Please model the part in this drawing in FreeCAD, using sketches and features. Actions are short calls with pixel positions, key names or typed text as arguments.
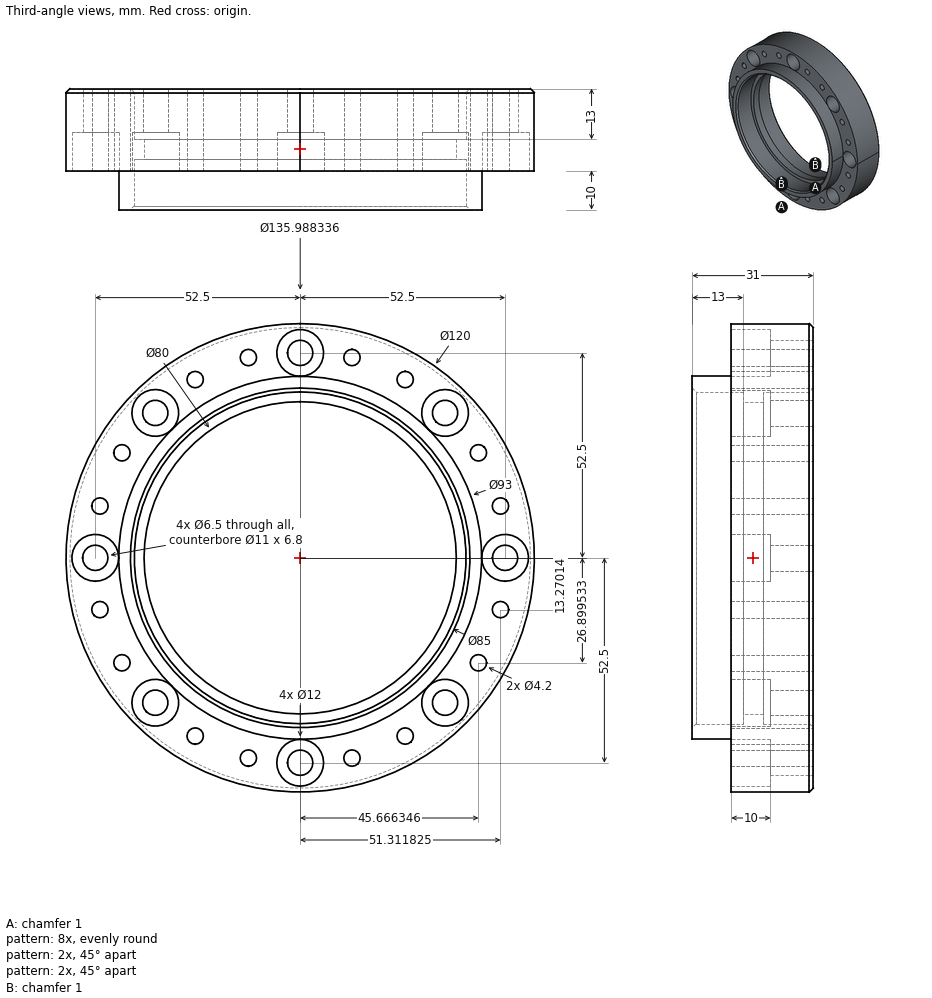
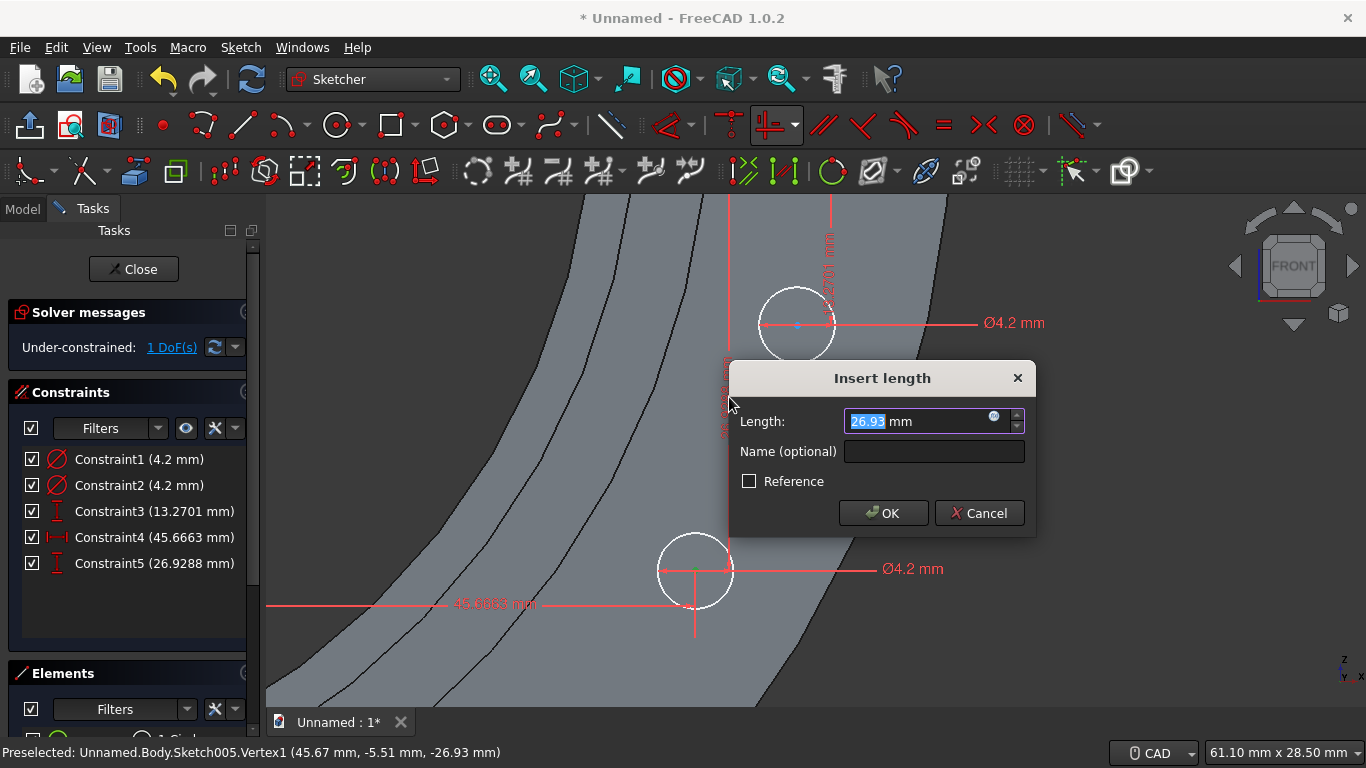
text(26.899533)
key(Return)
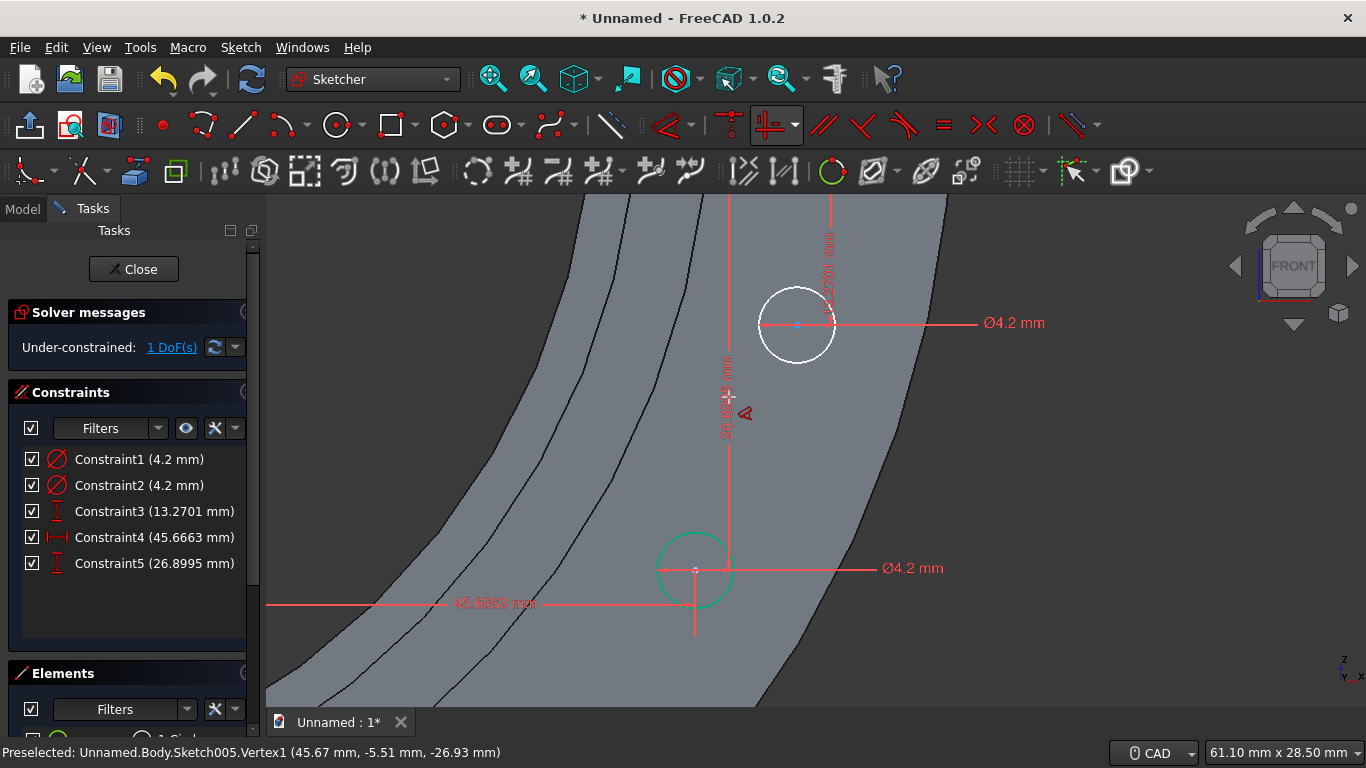
click(797, 325)
click(545, 359)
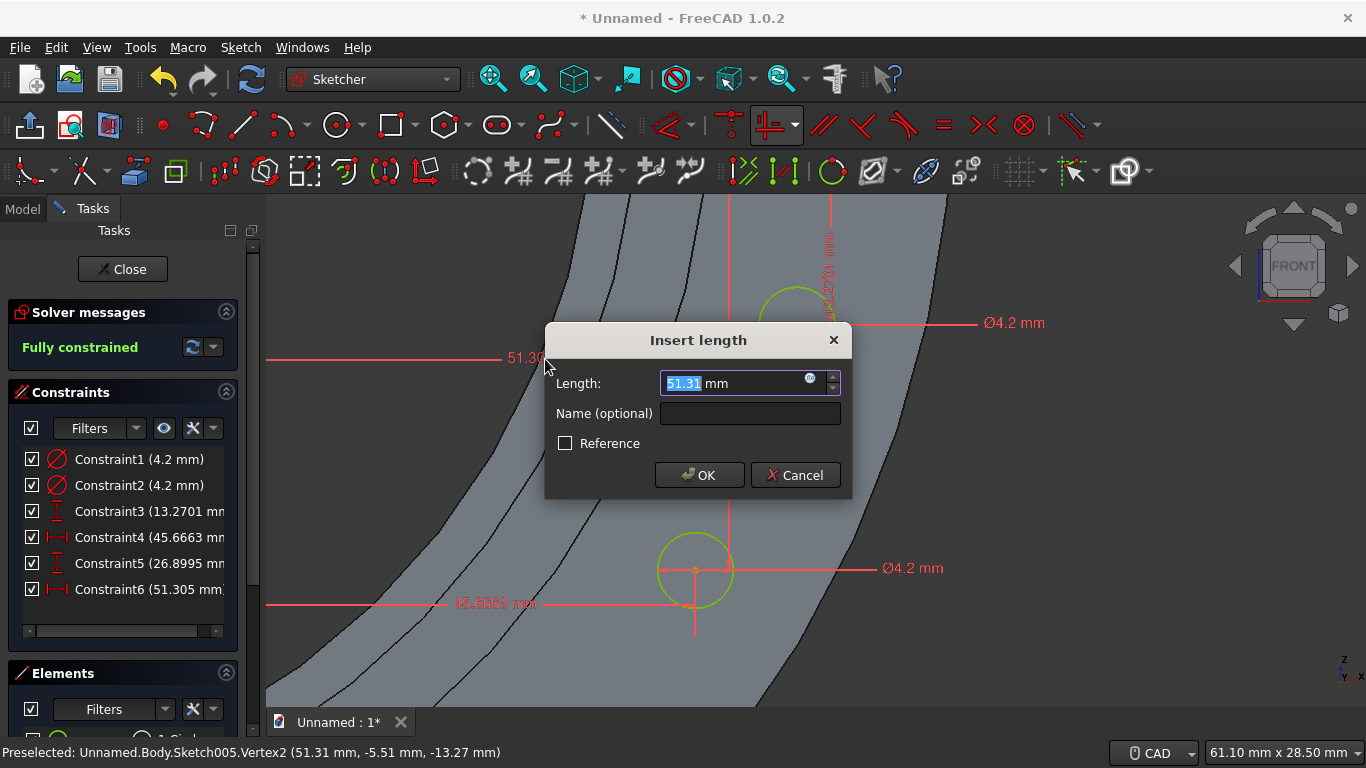
text(51.311825)
key(Return)
key(Escape)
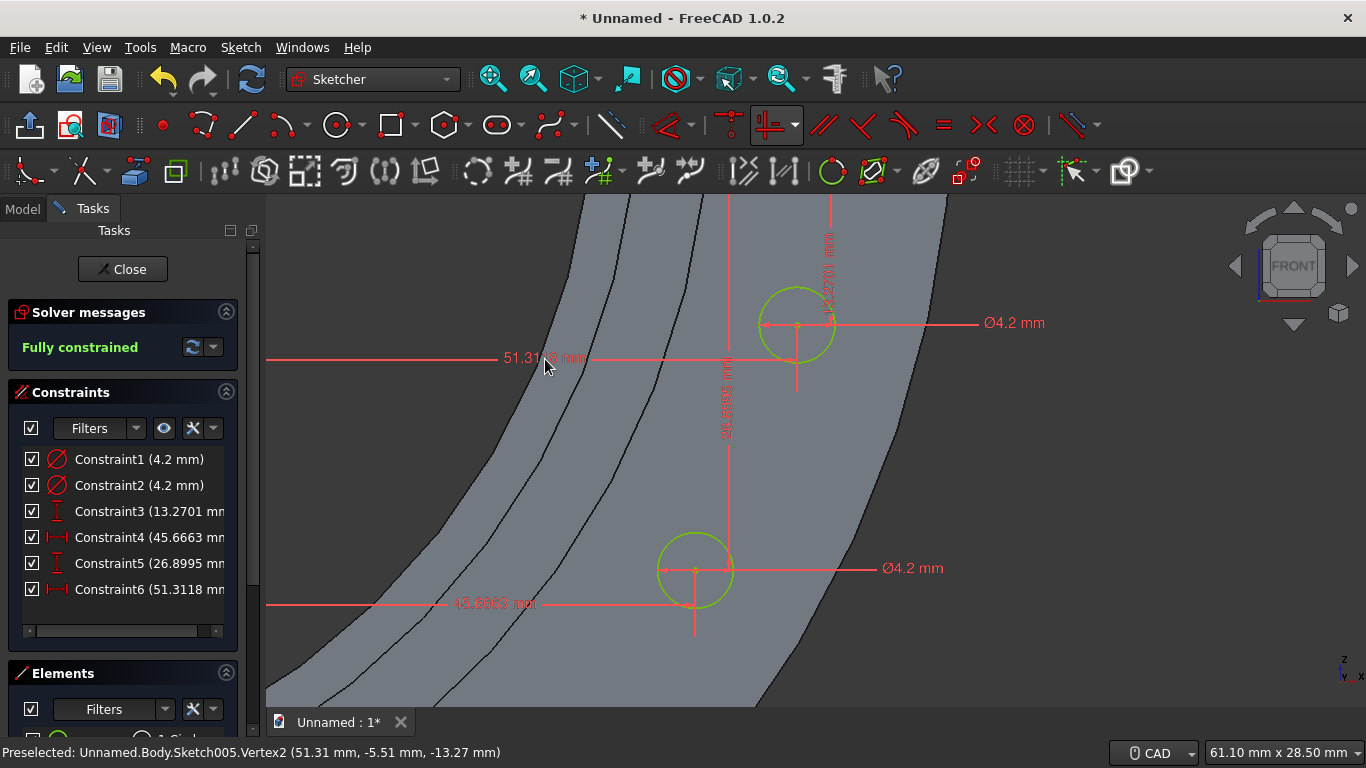
click(123, 269)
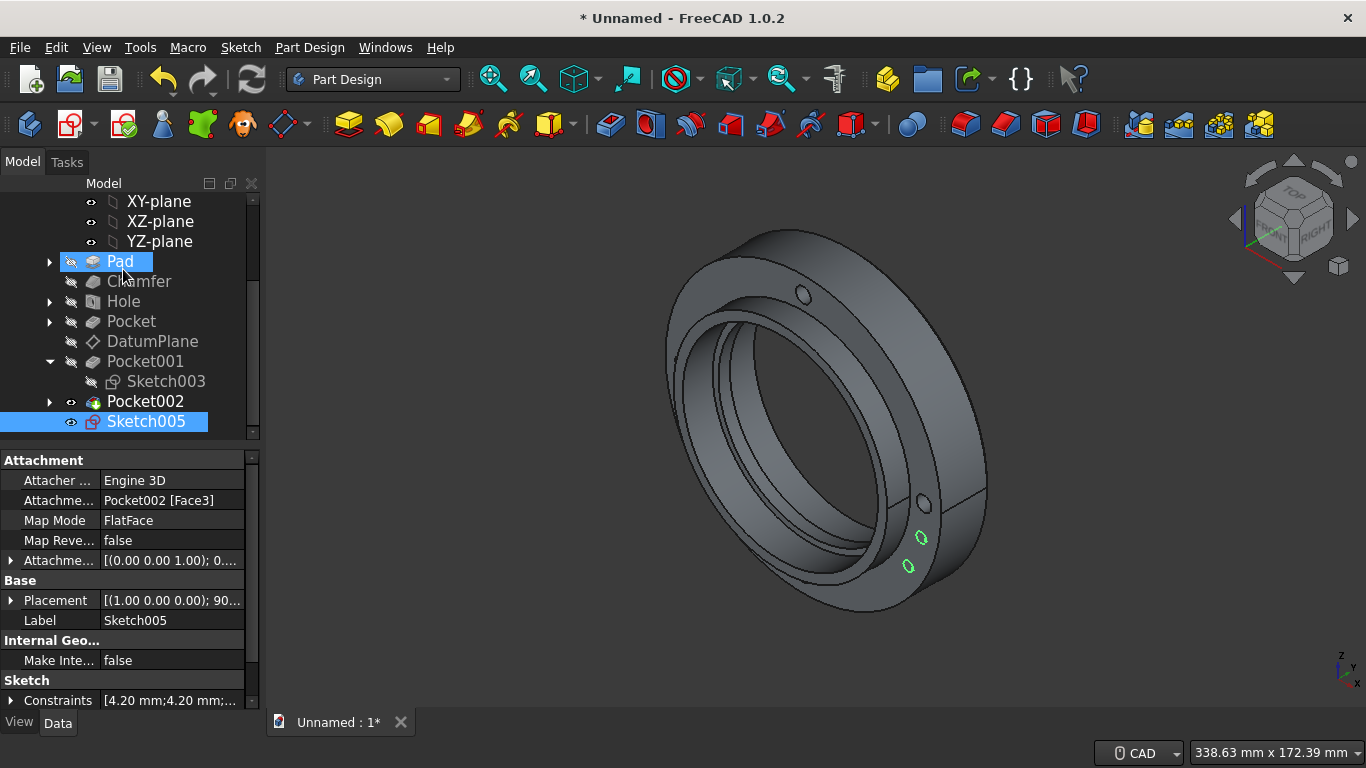
click(612, 124)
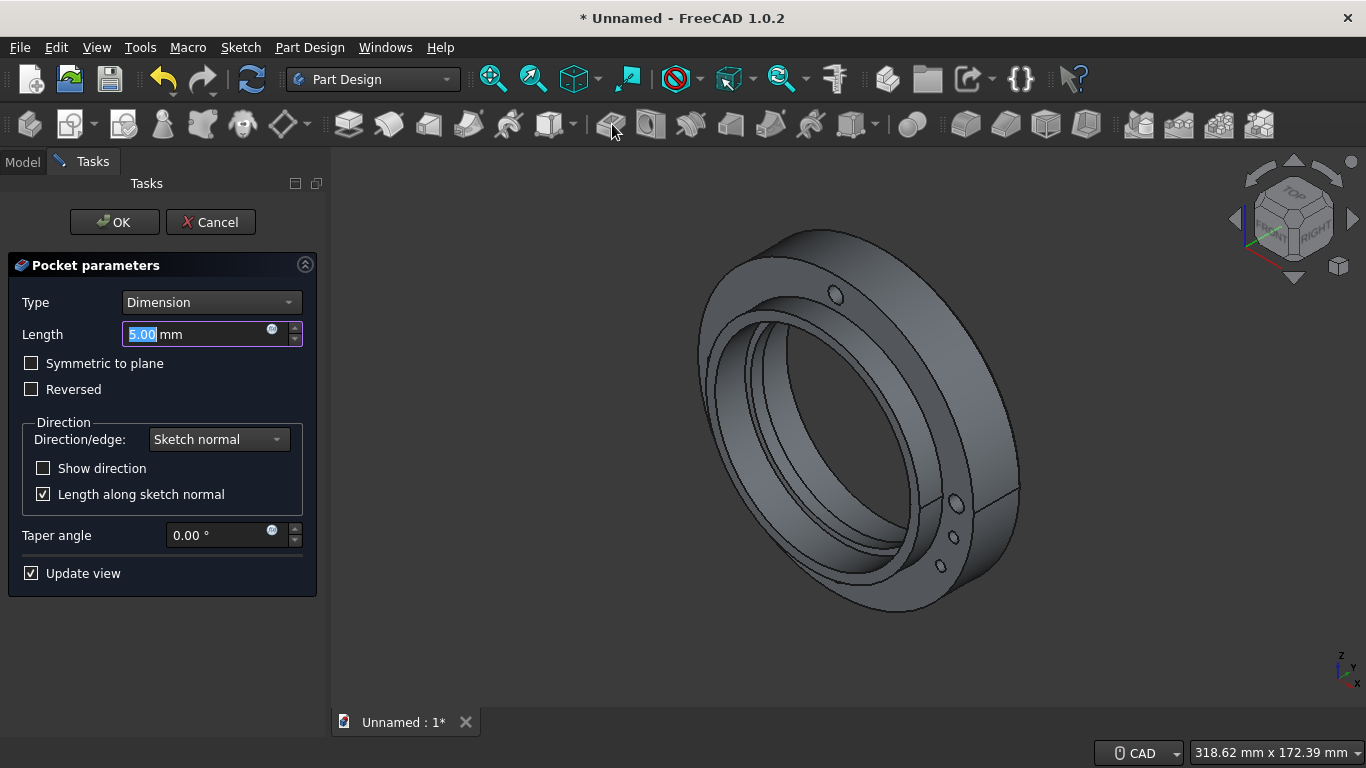
click(212, 302)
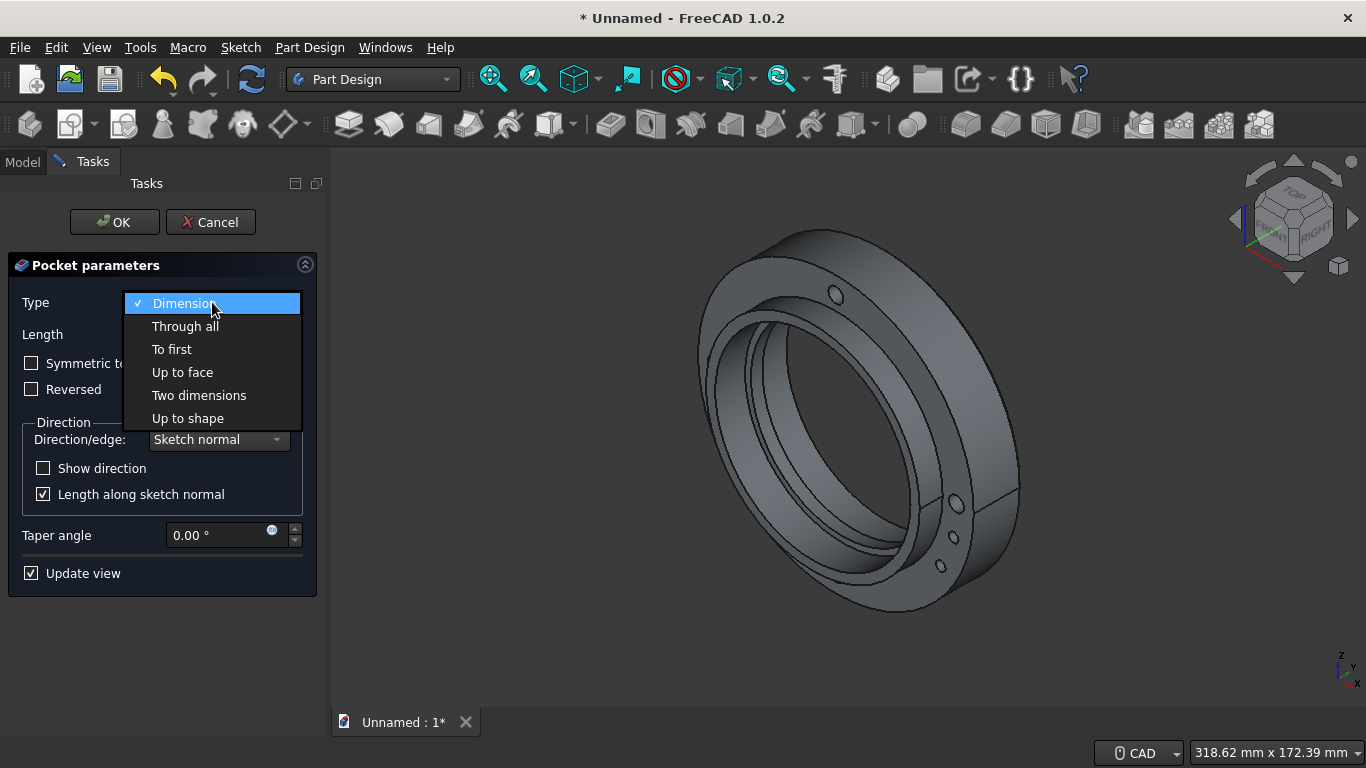
click(212, 326)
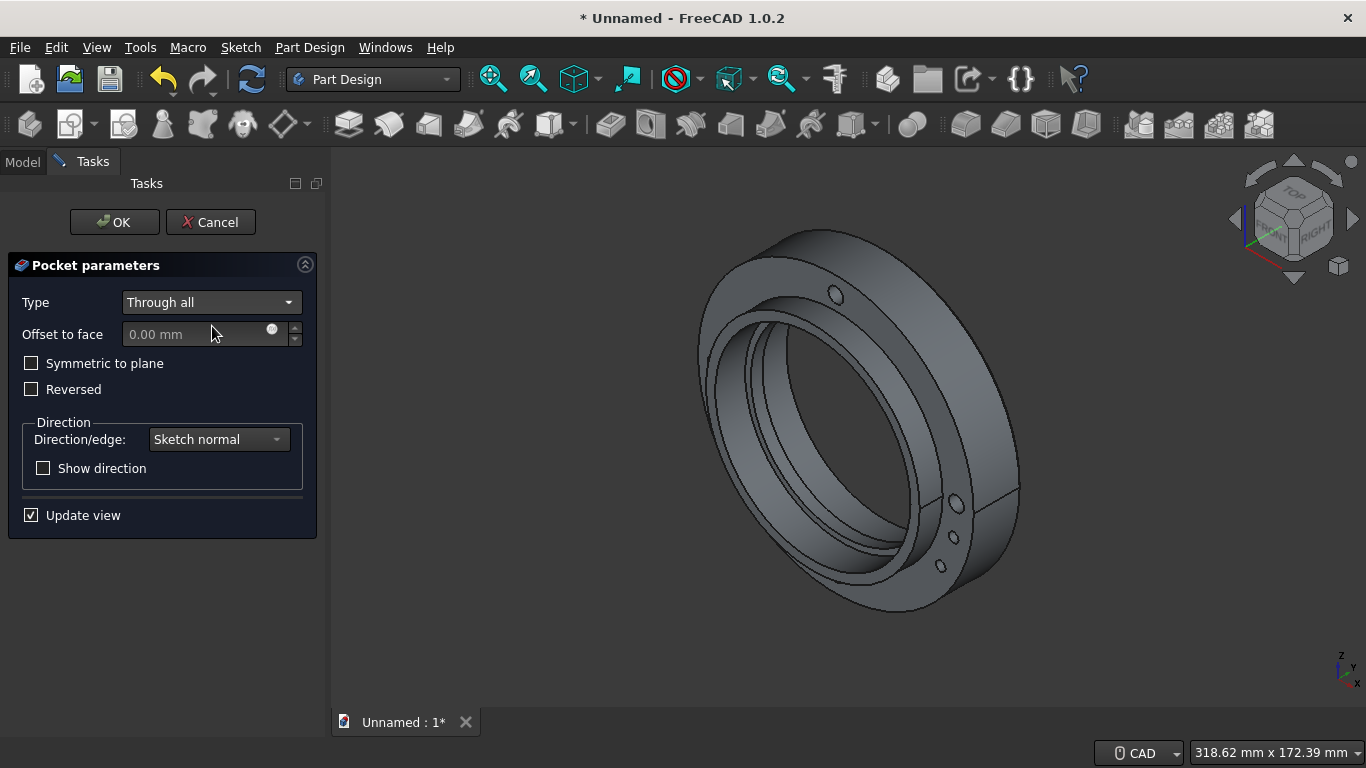
click(115, 222)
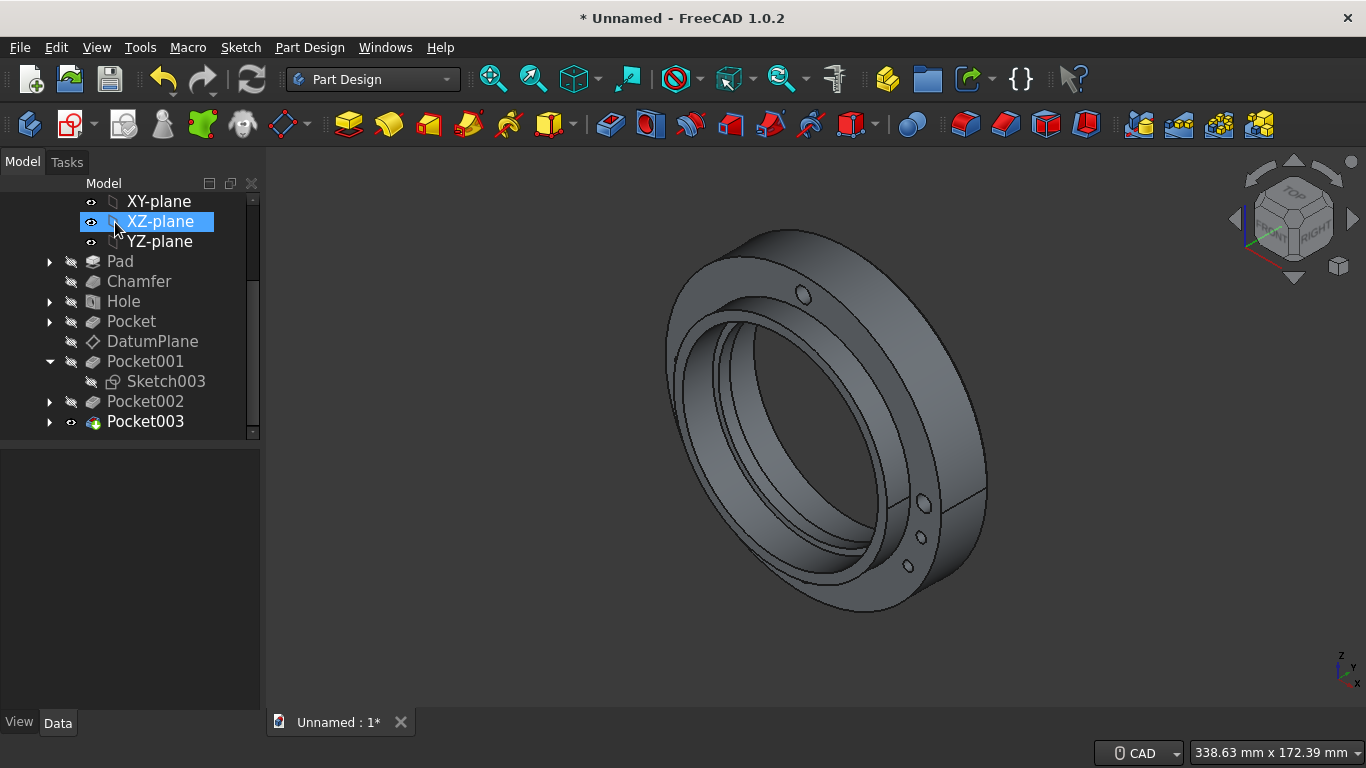
click(116, 422)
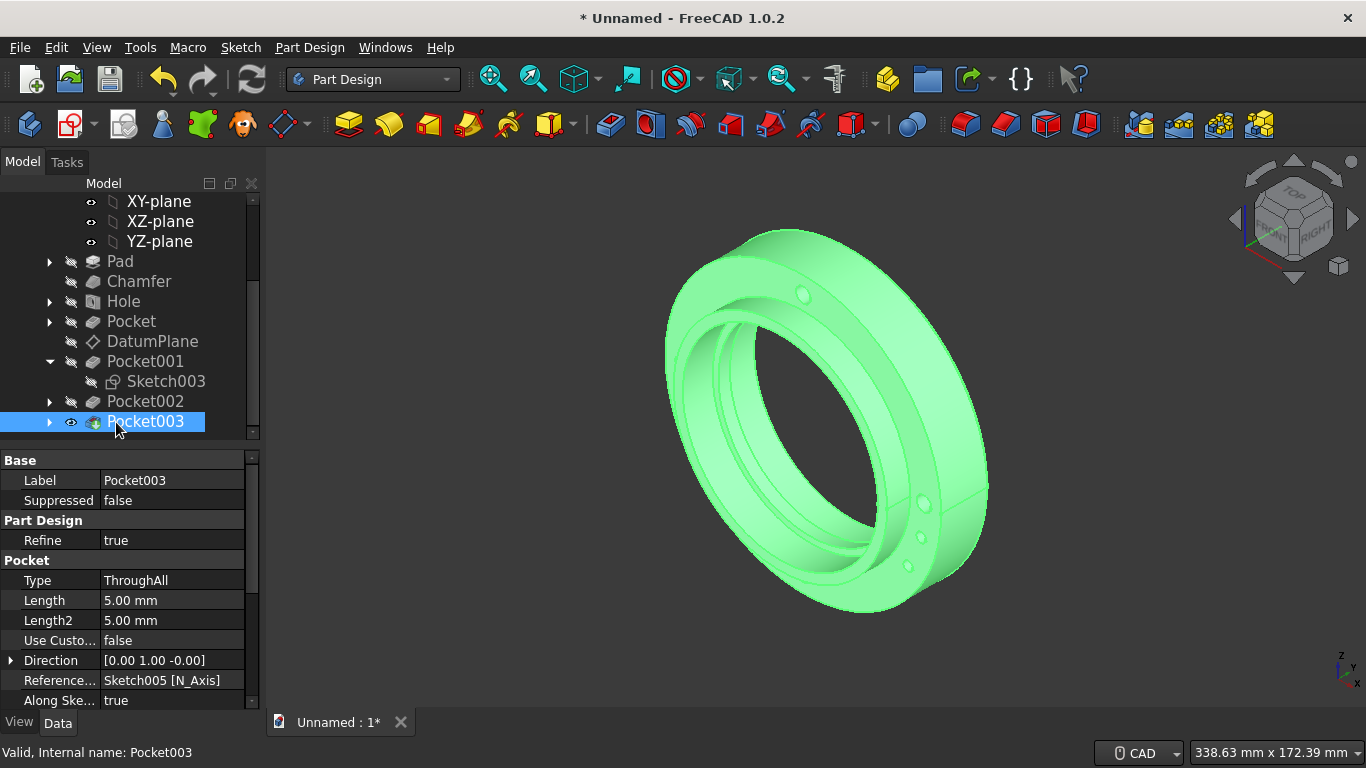
click(1220, 124)